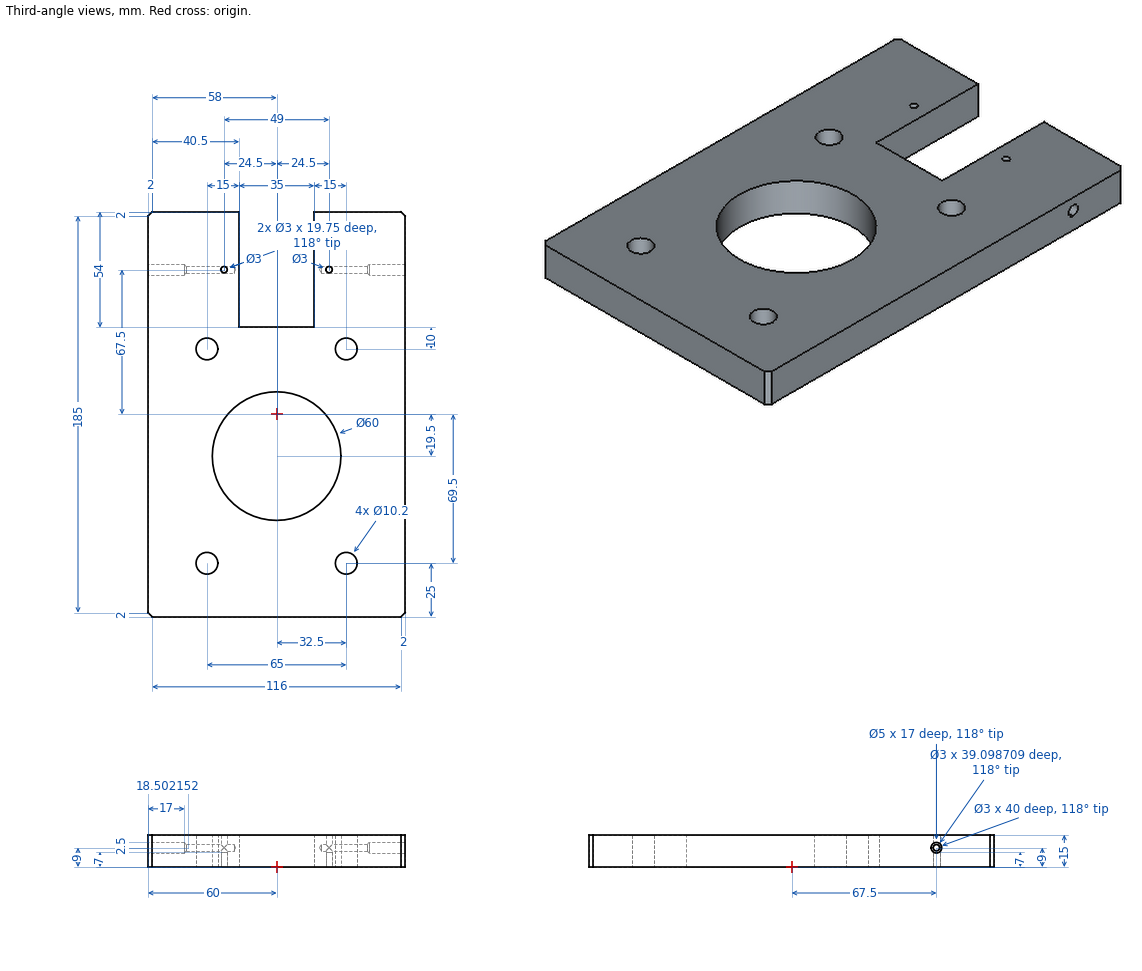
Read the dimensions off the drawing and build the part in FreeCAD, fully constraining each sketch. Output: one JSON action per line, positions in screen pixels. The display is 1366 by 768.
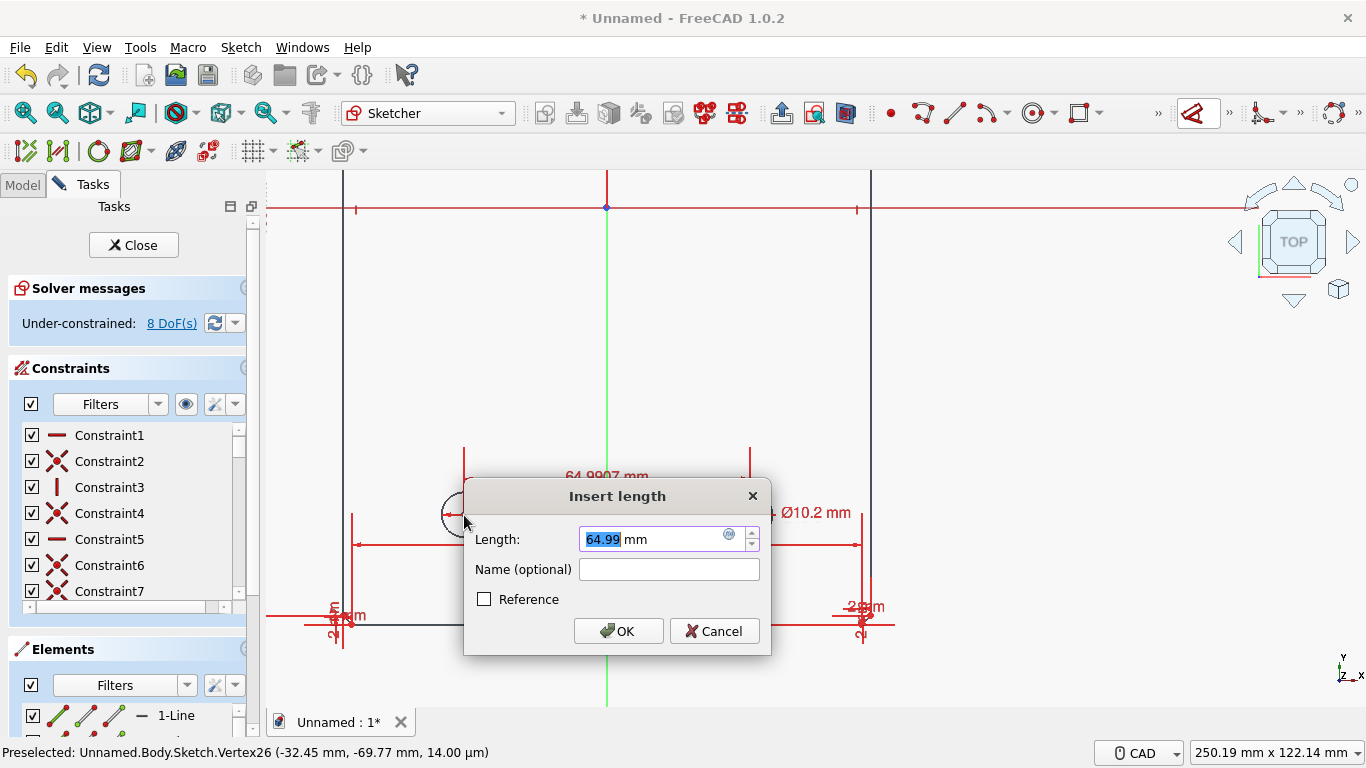
{"action": "type", "text": "65"}
{"action": "key", "text": "Return"}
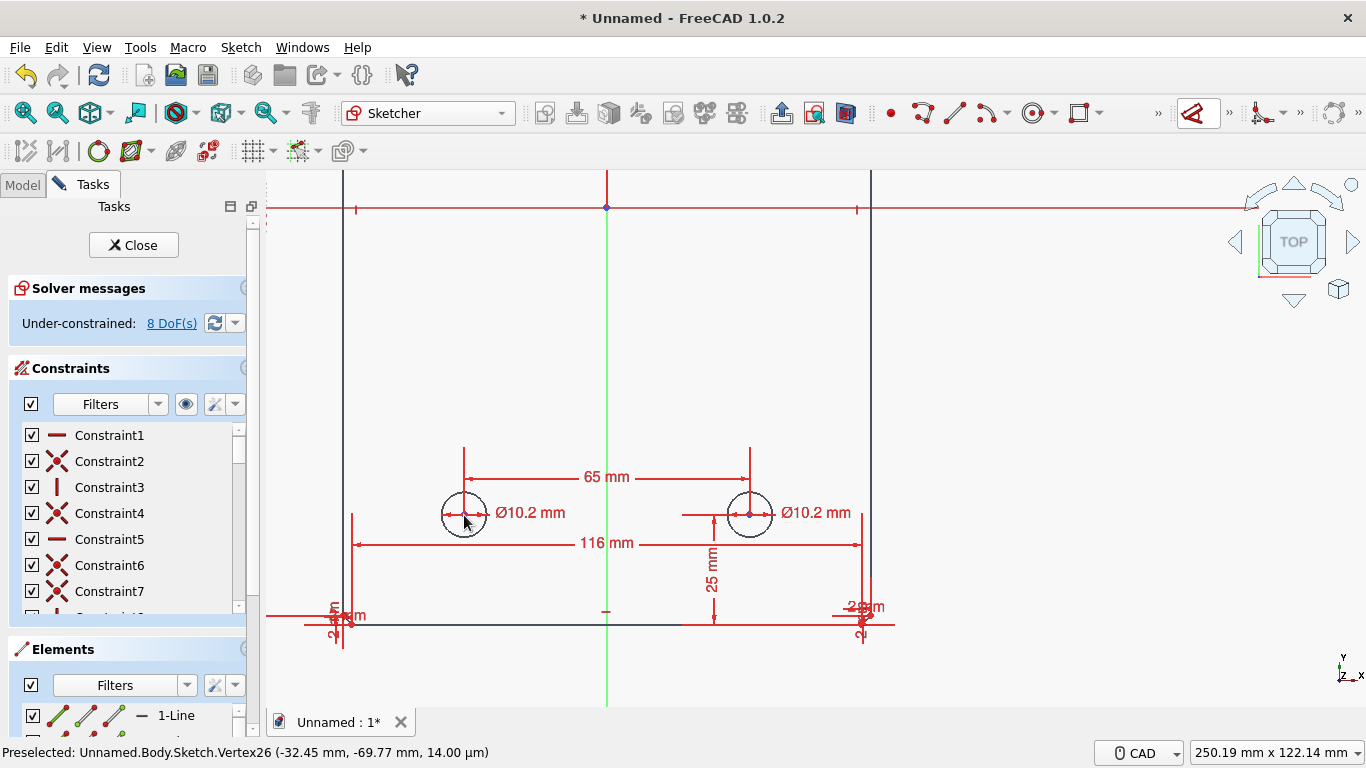
{"action": "left_click", "coordinate": [352, 625]}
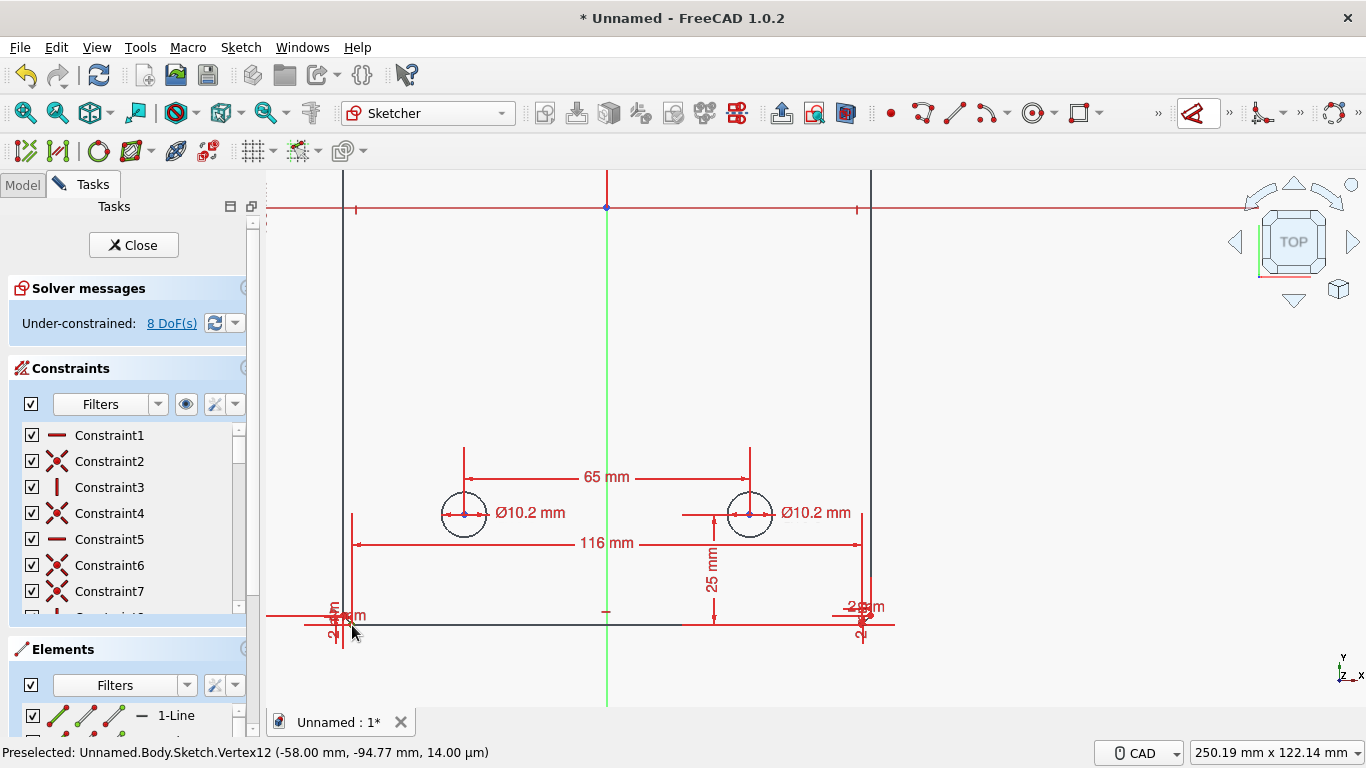
{"action": "left_click", "coordinate": [464, 515]}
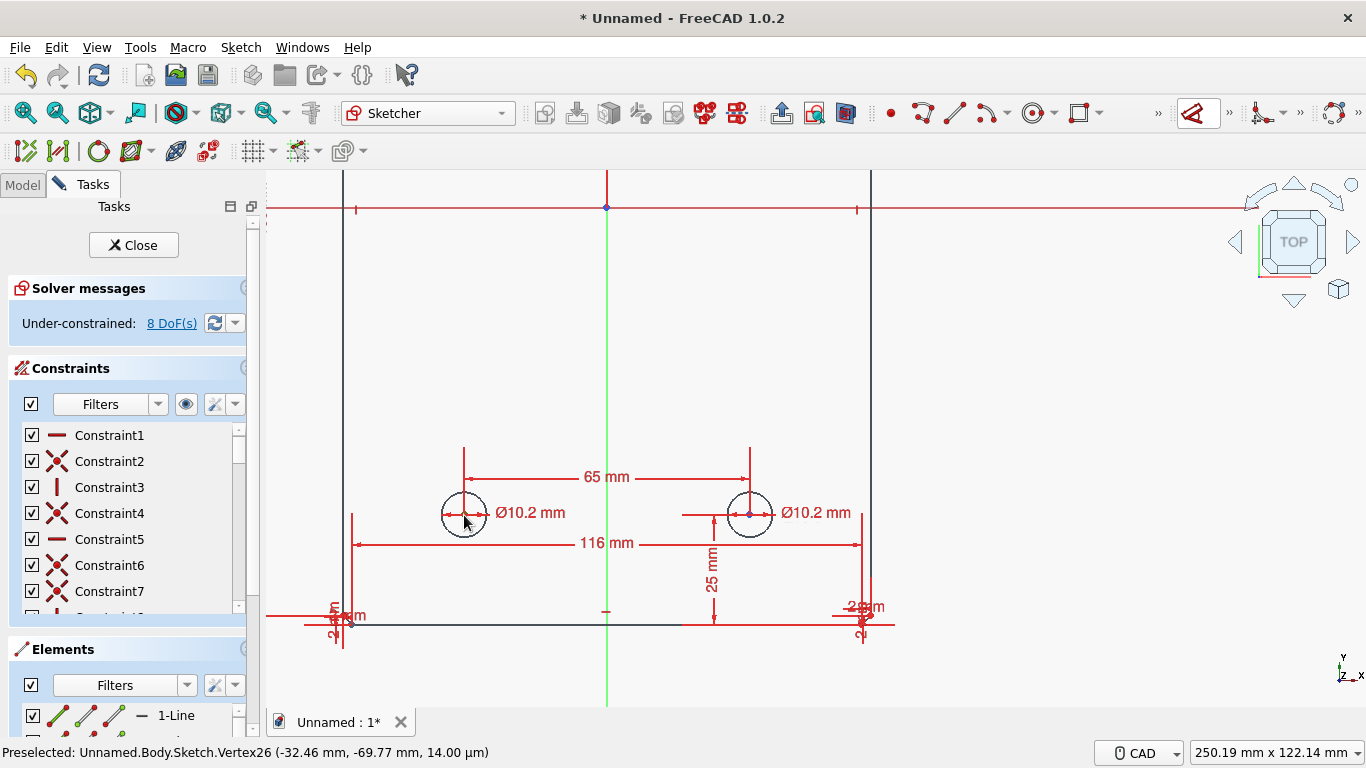
{"action": "left_click", "coordinate": [1214, 114]}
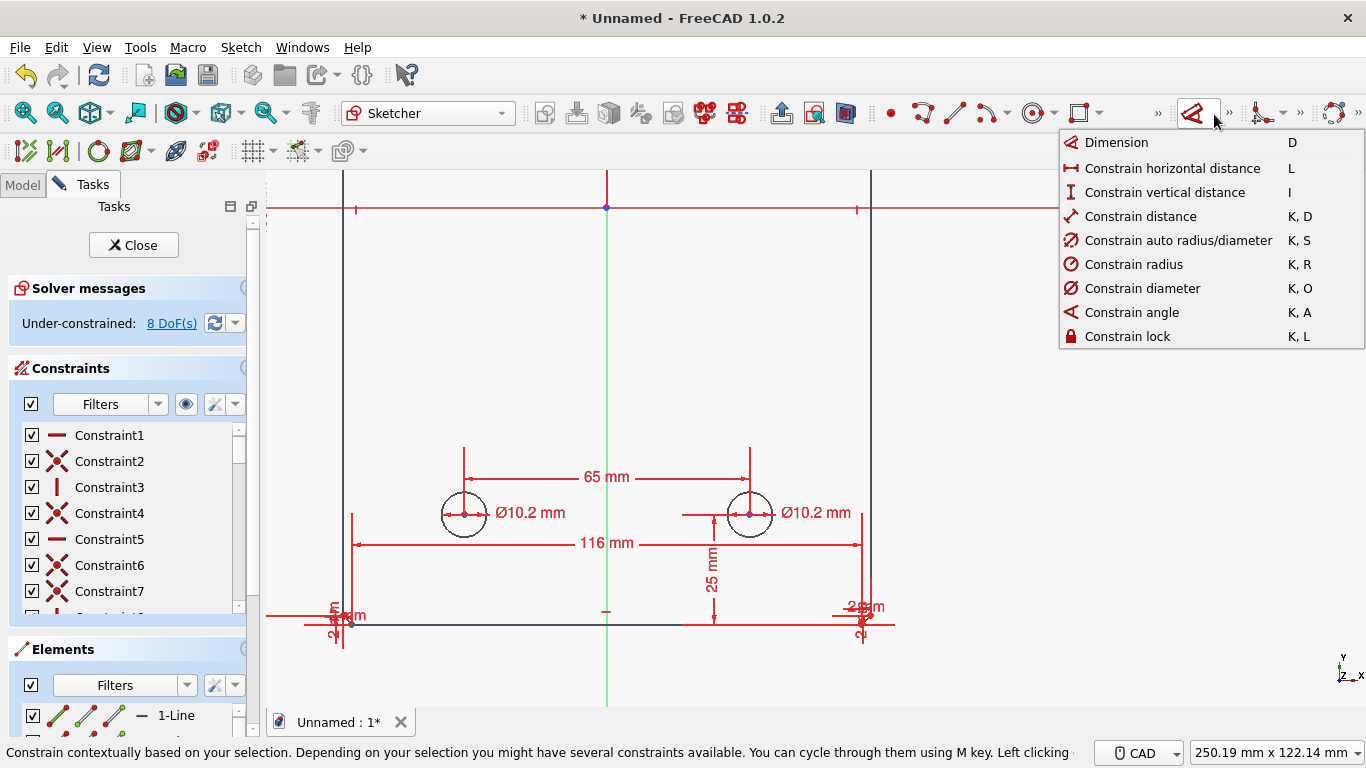
{"action": "left_click", "coordinate": [1212, 192]}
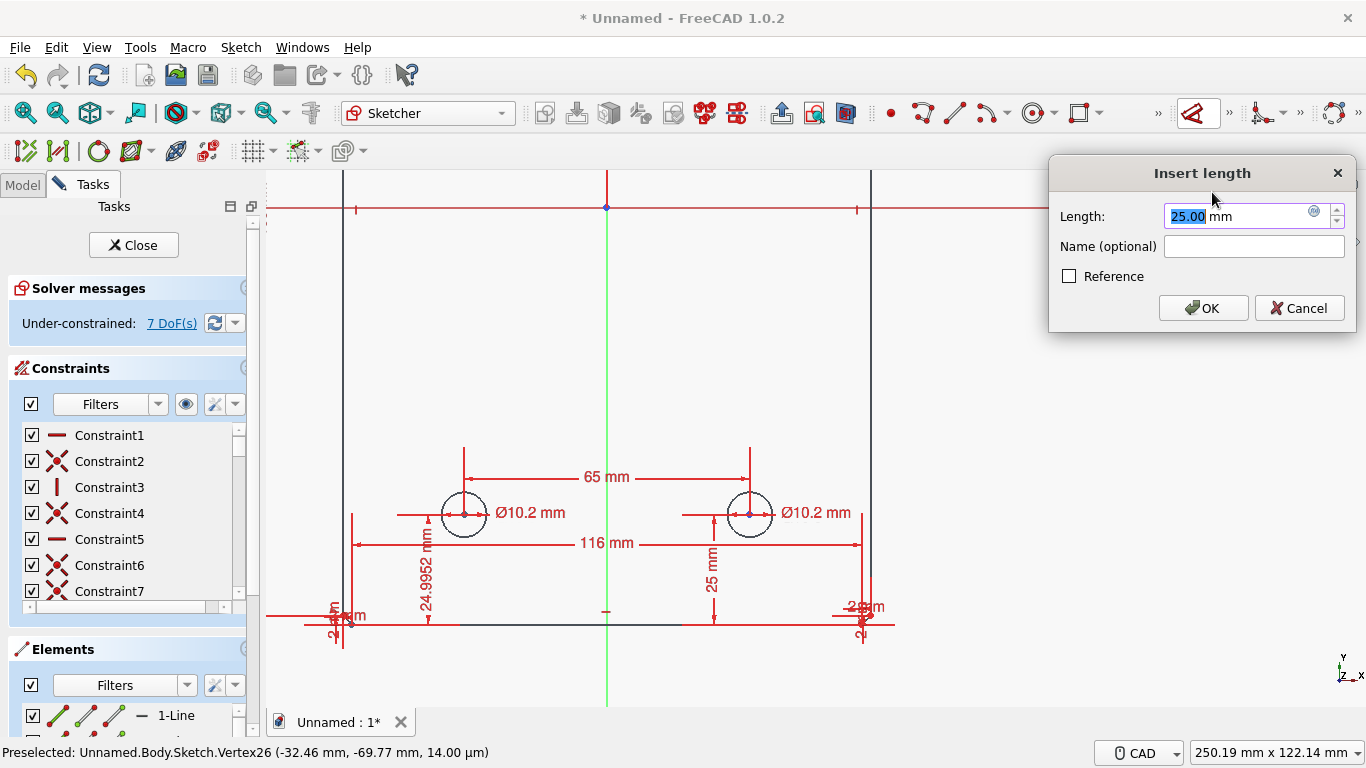
{"action": "type", "text": "25"}
{"action": "key", "text": "Return"}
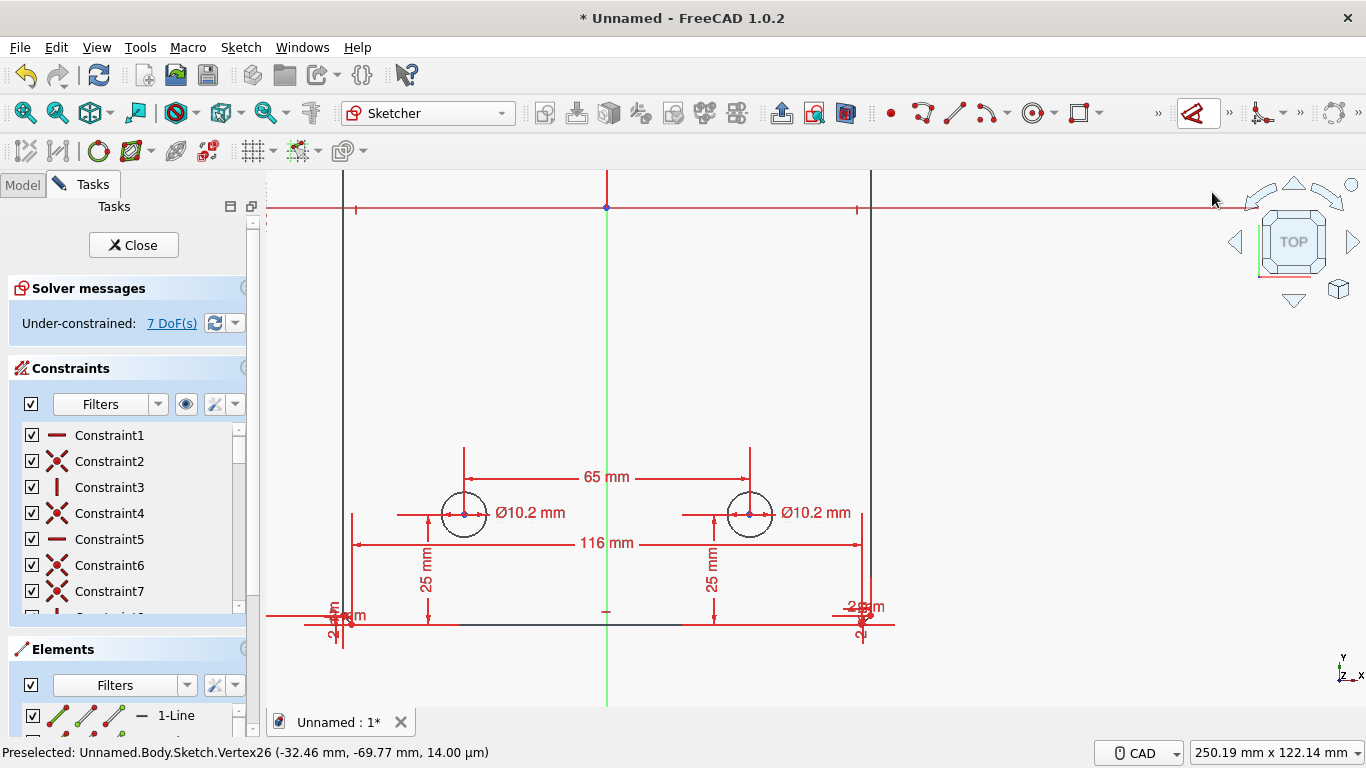
{"action": "scroll", "coordinate": [862, 627], "scroll_direction": "down", "scroll_amount": 4}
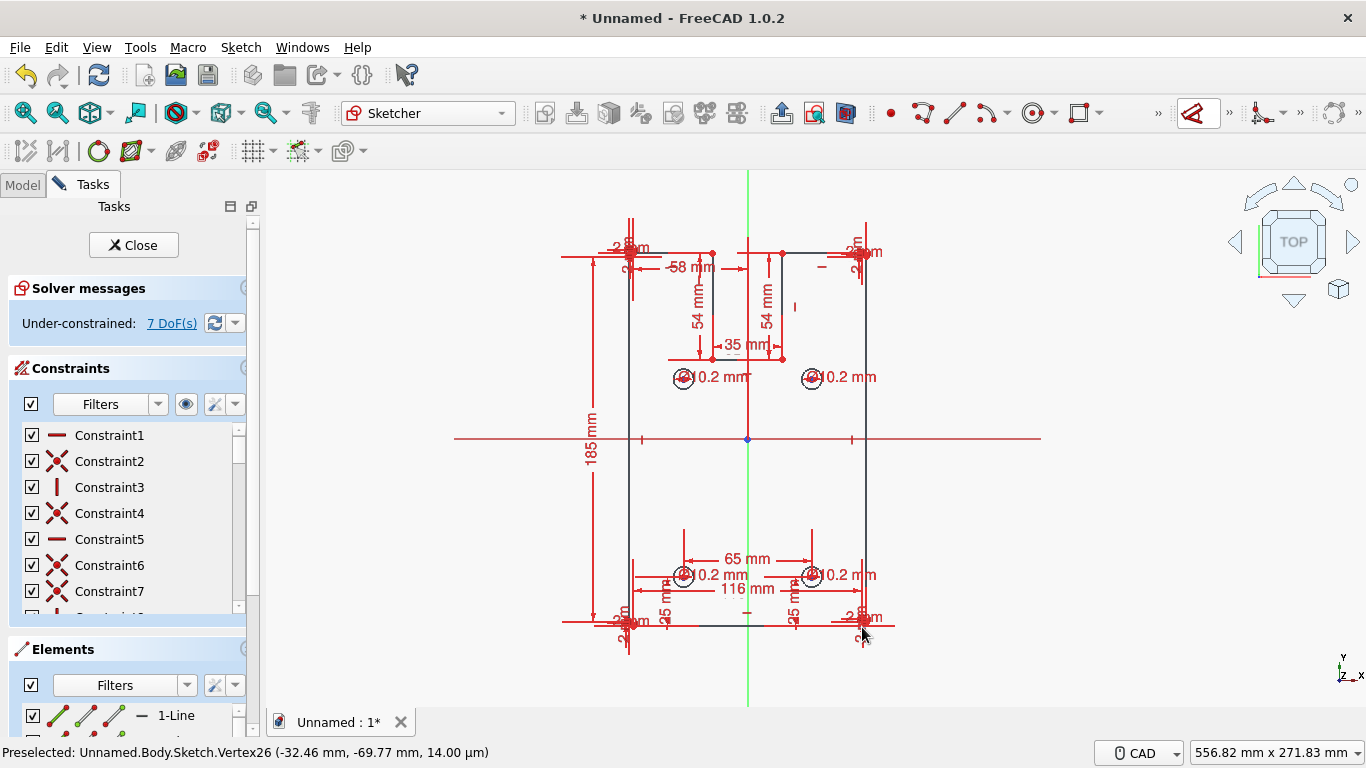
{"action": "scroll", "coordinate": [782, 360], "scroll_direction": "up", "scroll_amount": 2}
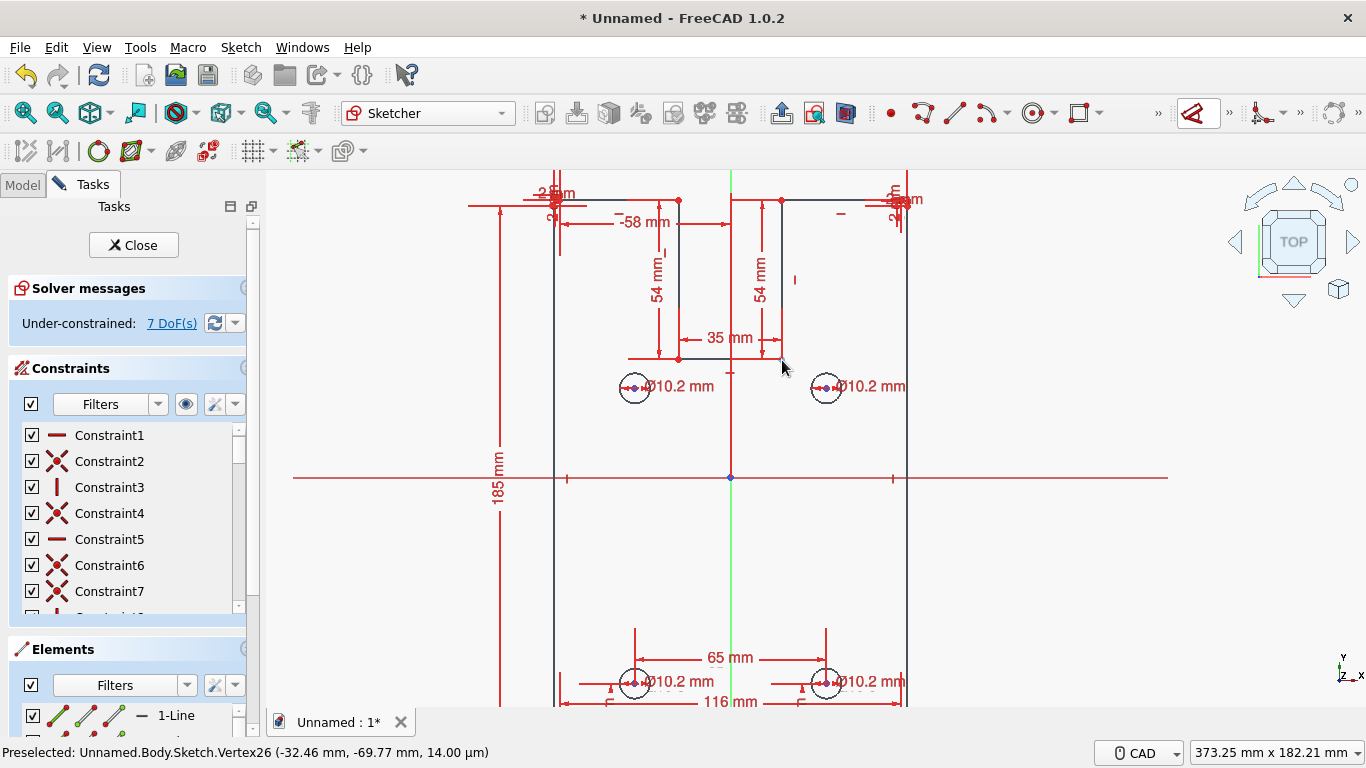
{"action": "left_click", "coordinate": [782, 359]}